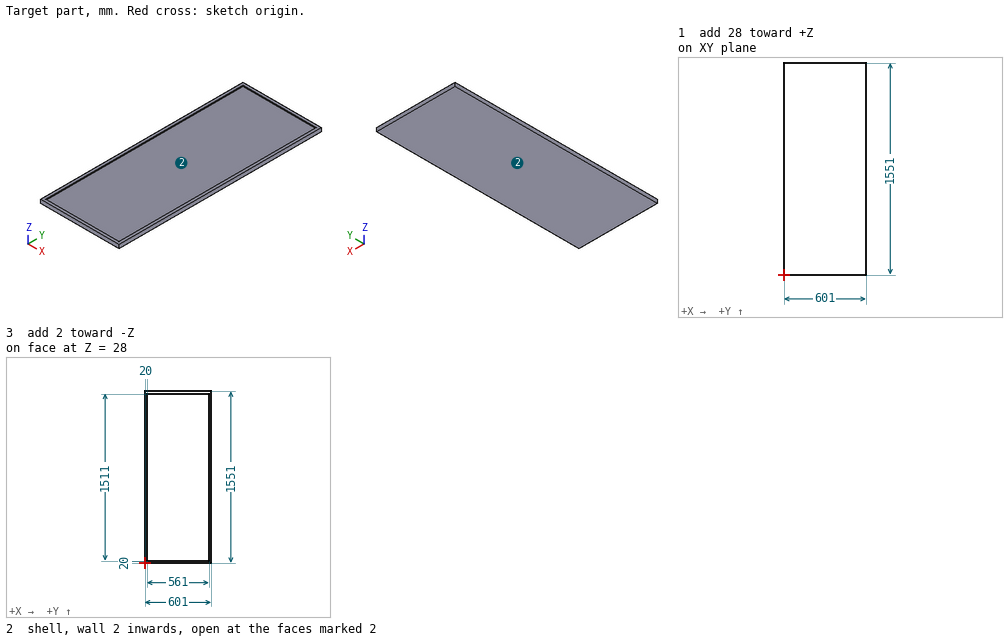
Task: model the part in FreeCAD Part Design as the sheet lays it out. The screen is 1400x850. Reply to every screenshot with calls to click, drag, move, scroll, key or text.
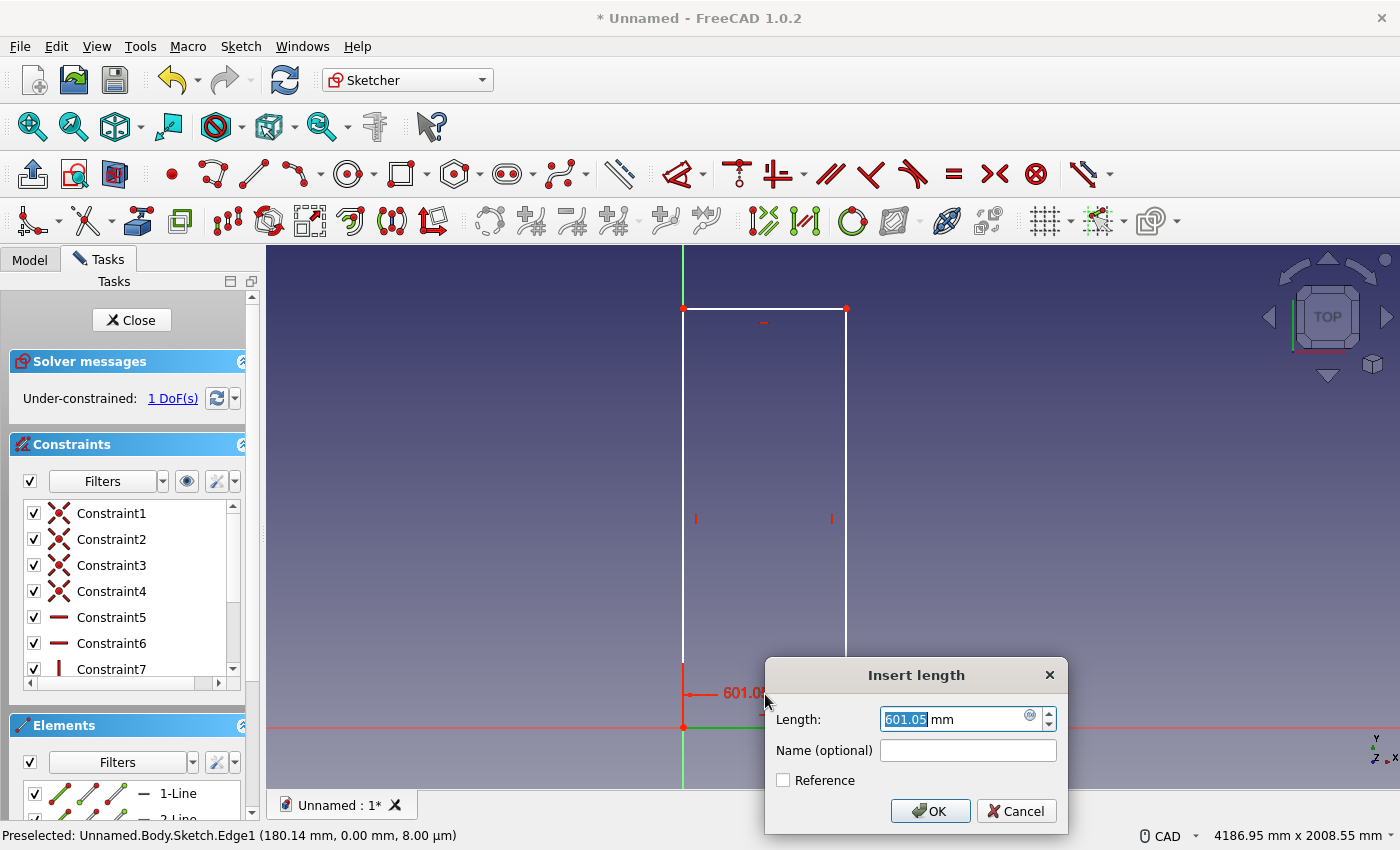
text(601)
key(Return)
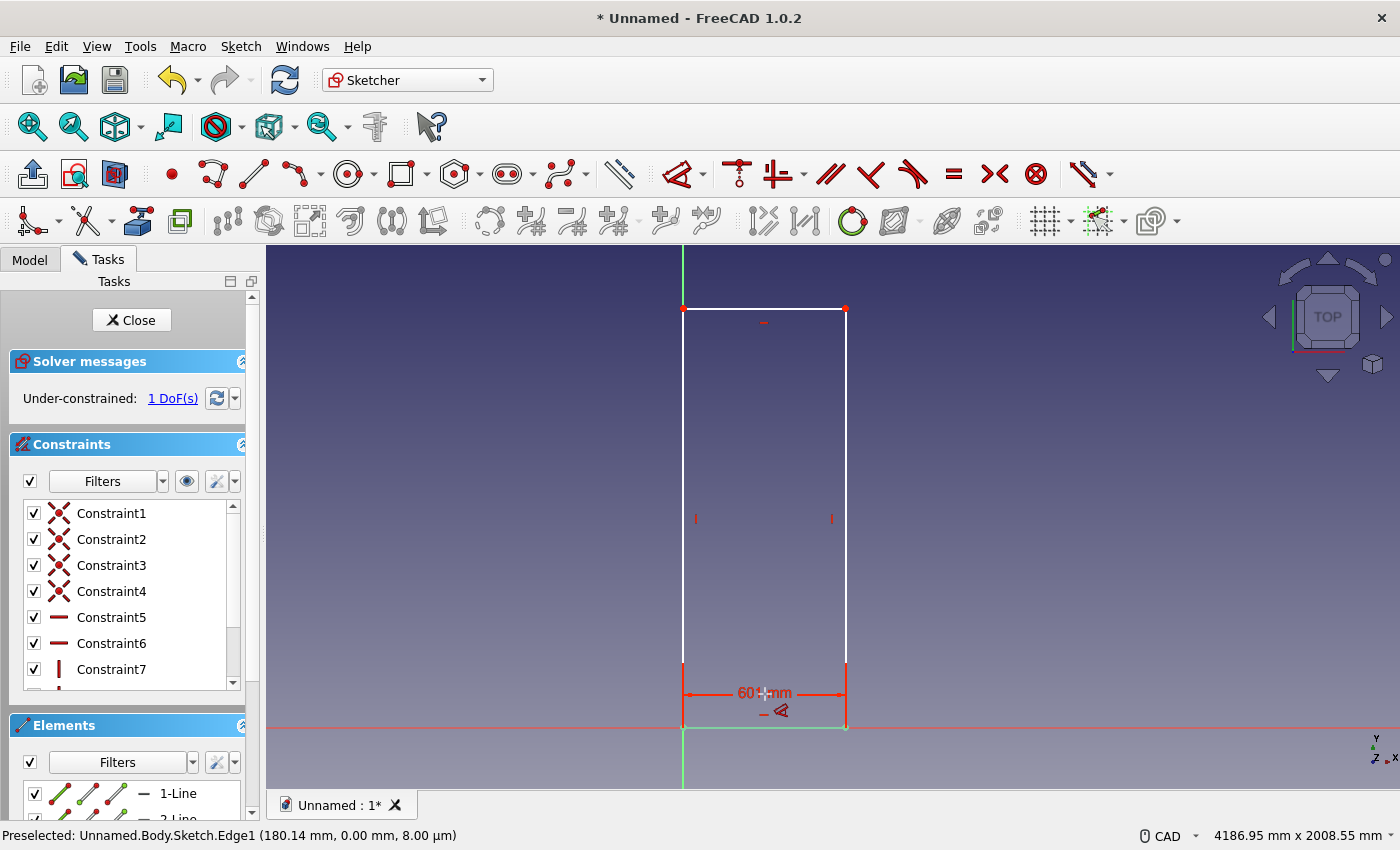
click(846, 602)
click(880, 518)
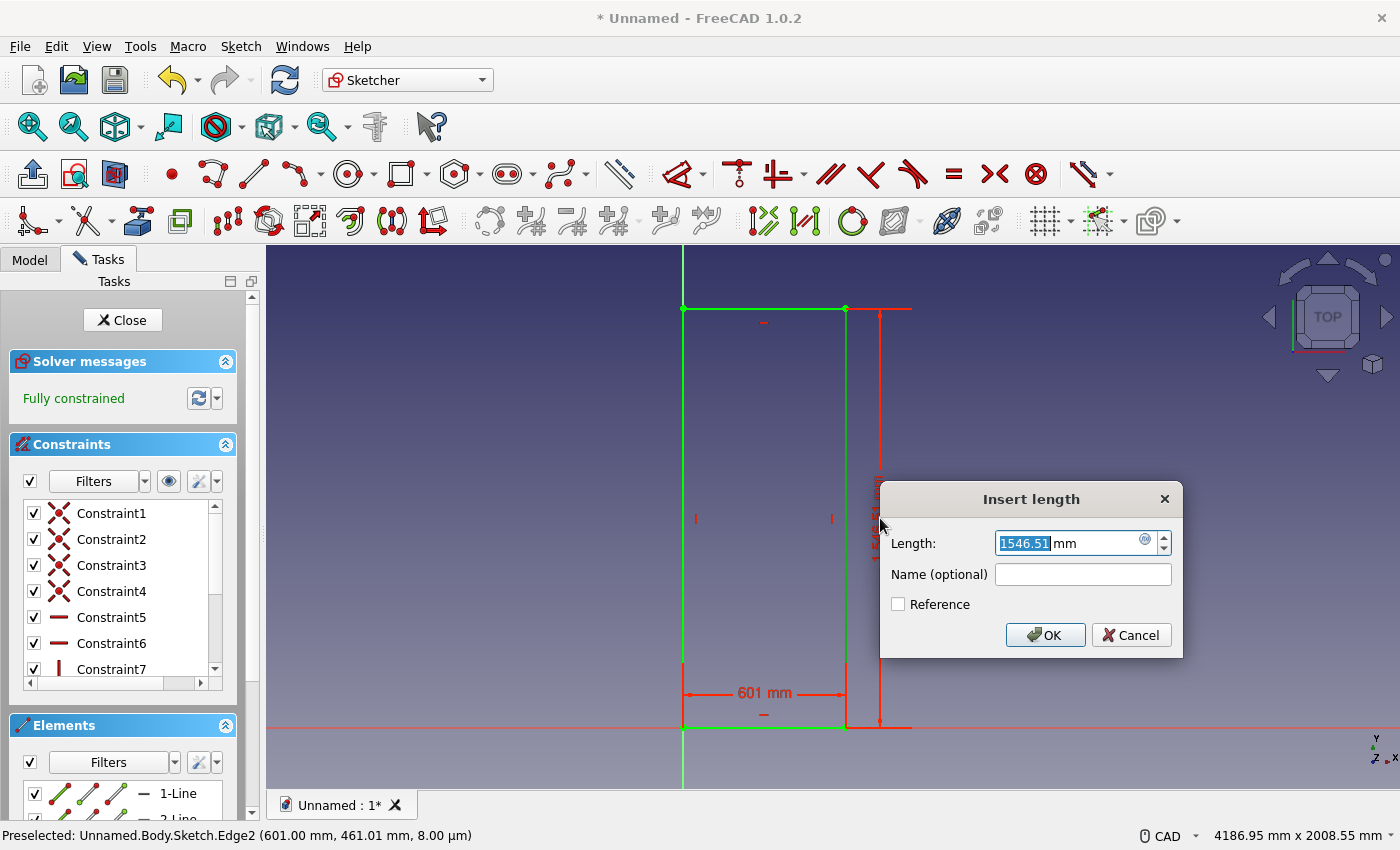
text(1551)
key(Return)
key(Escape)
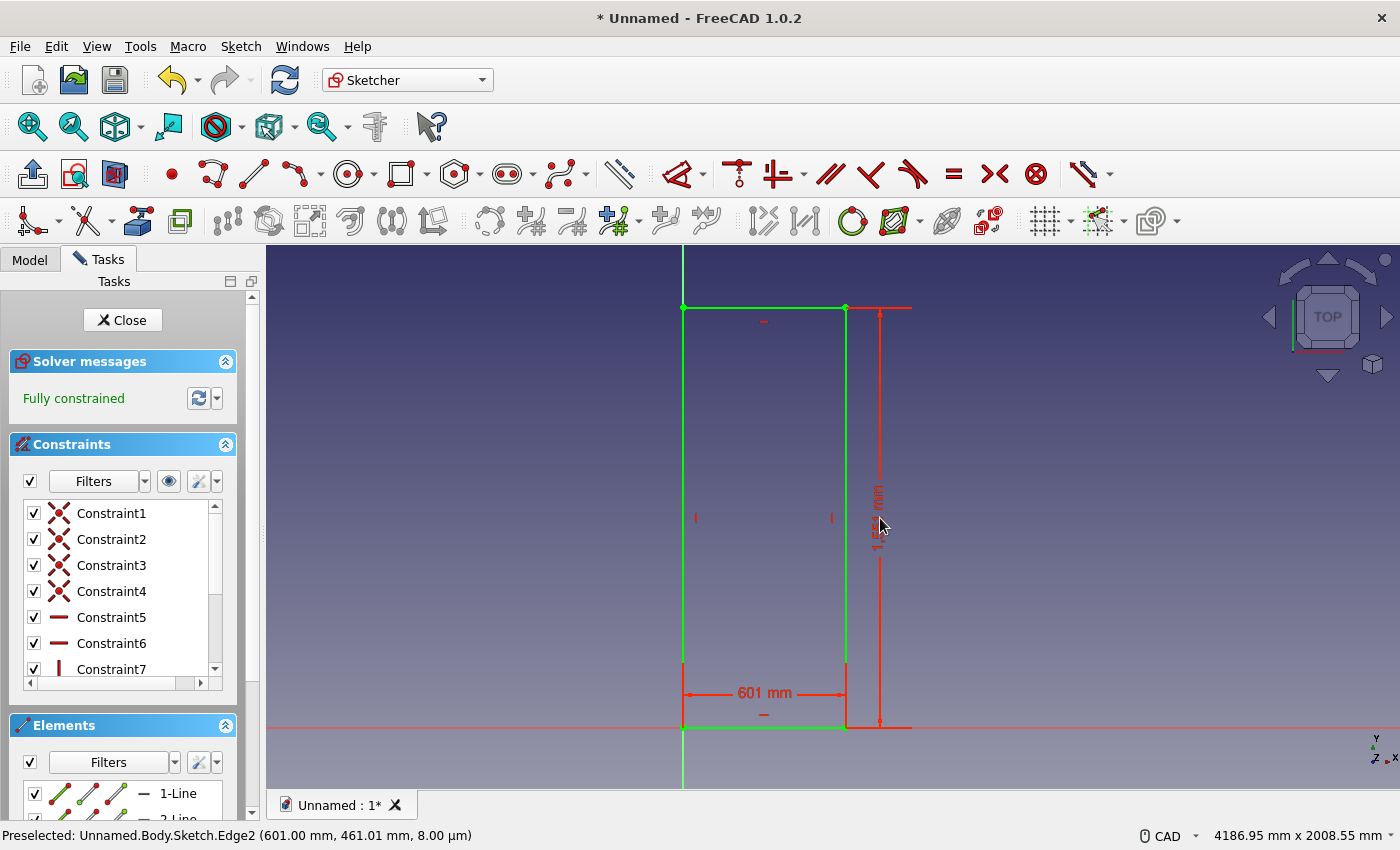
click(123, 320)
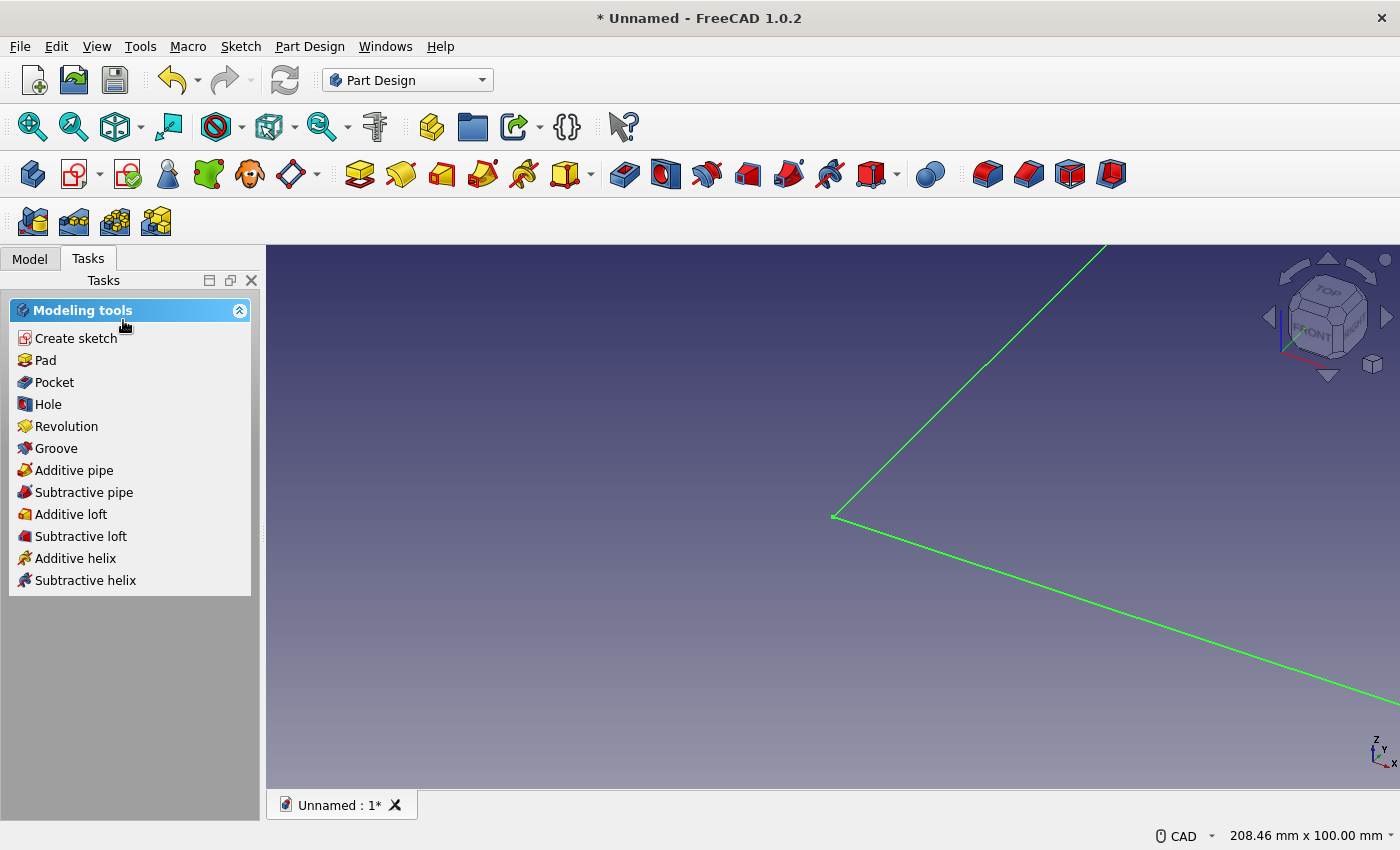
click(360, 174)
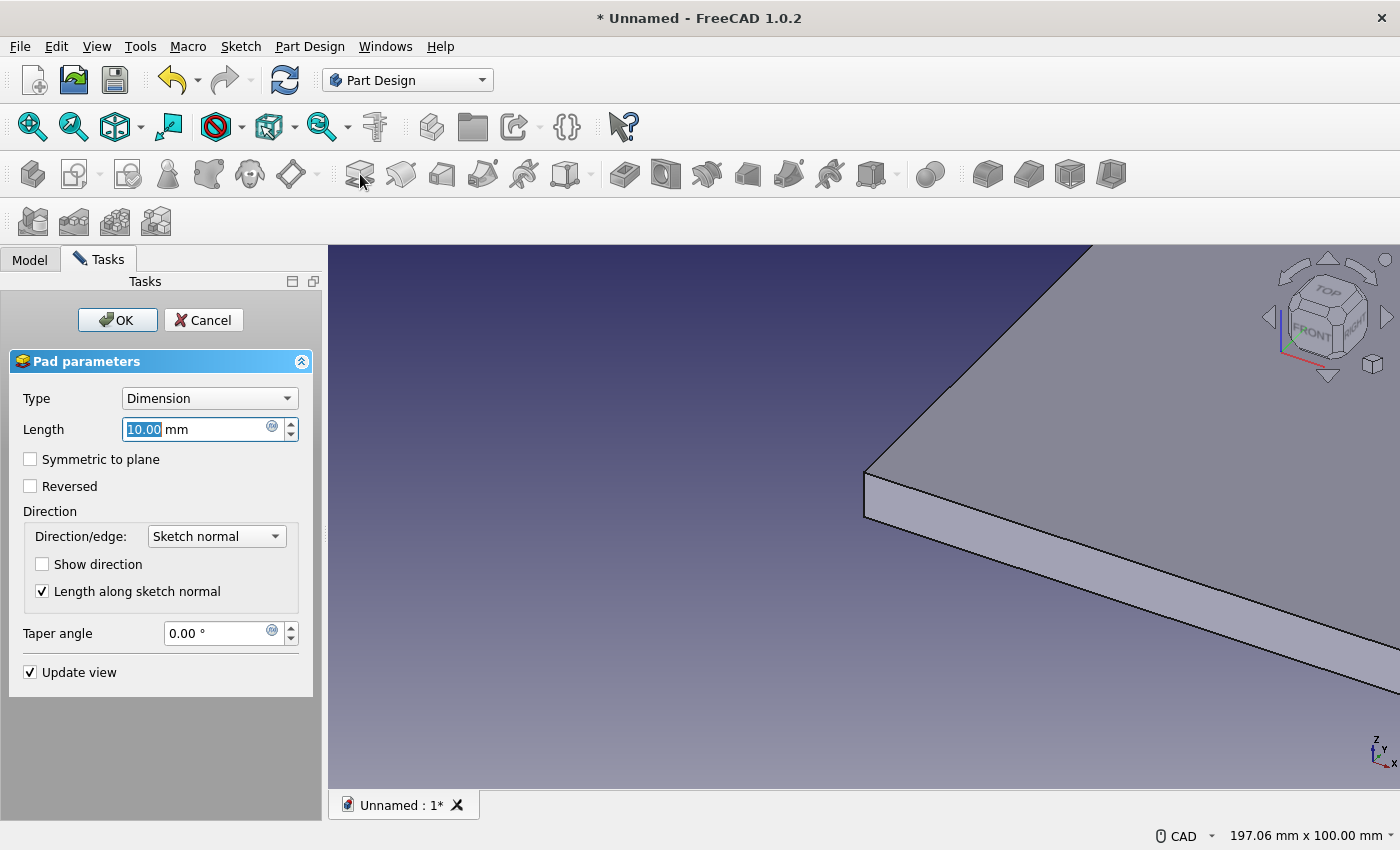
text(28)
key(Tab)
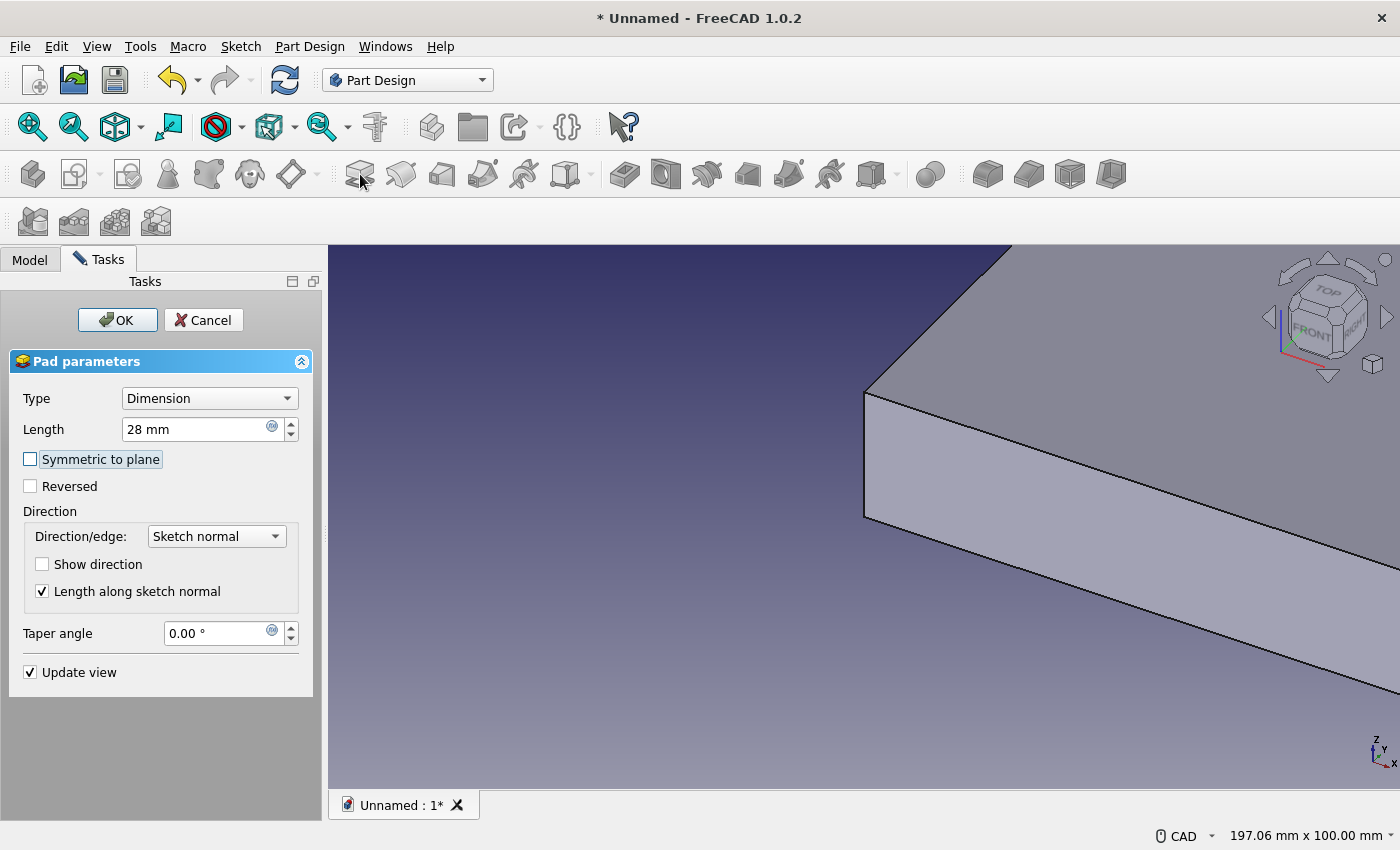
click(118, 320)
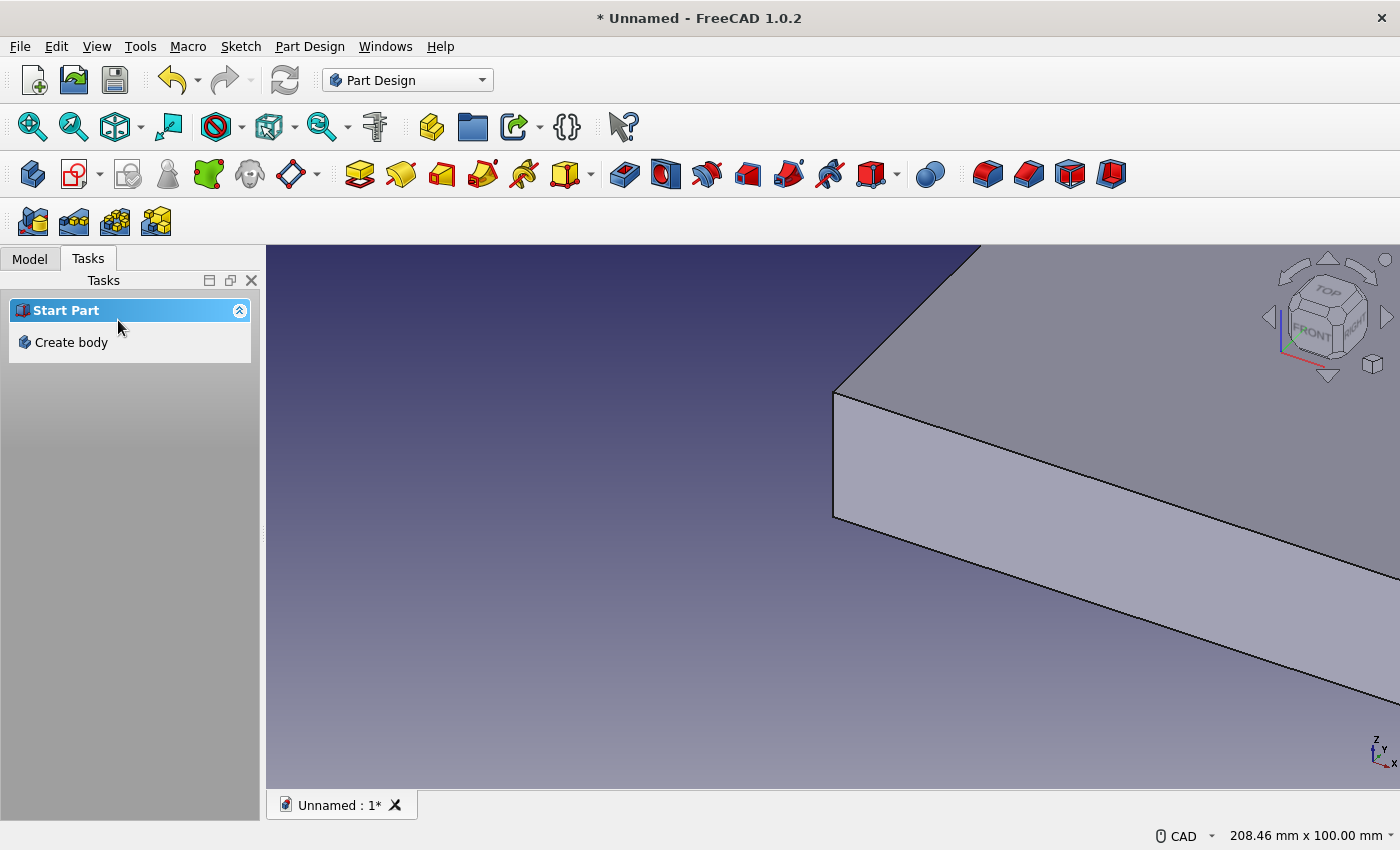
click(33, 128)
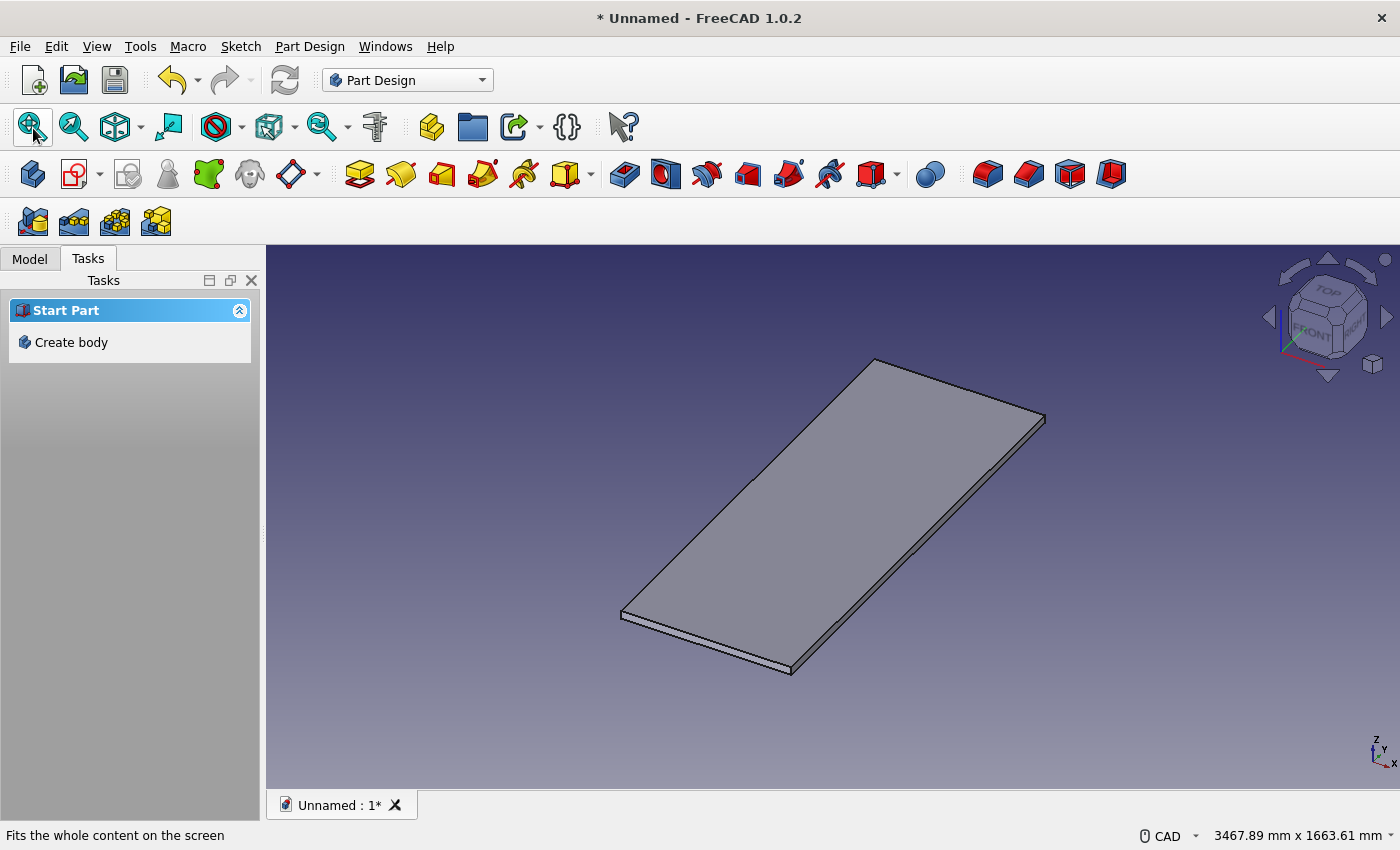
click(905, 440)